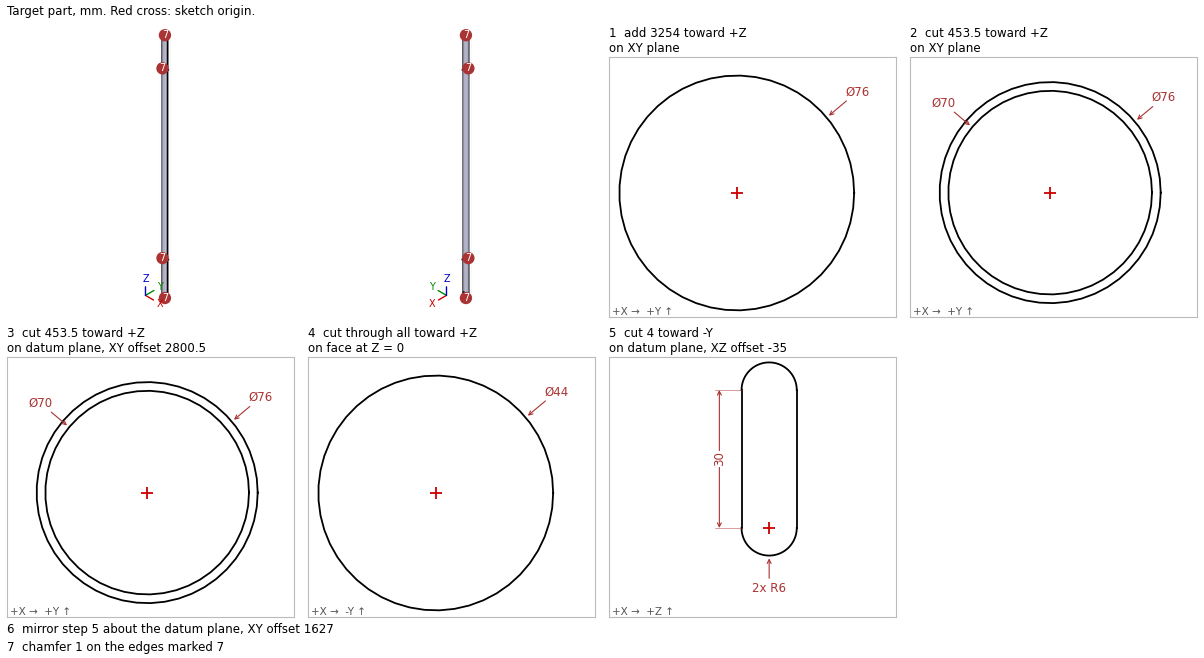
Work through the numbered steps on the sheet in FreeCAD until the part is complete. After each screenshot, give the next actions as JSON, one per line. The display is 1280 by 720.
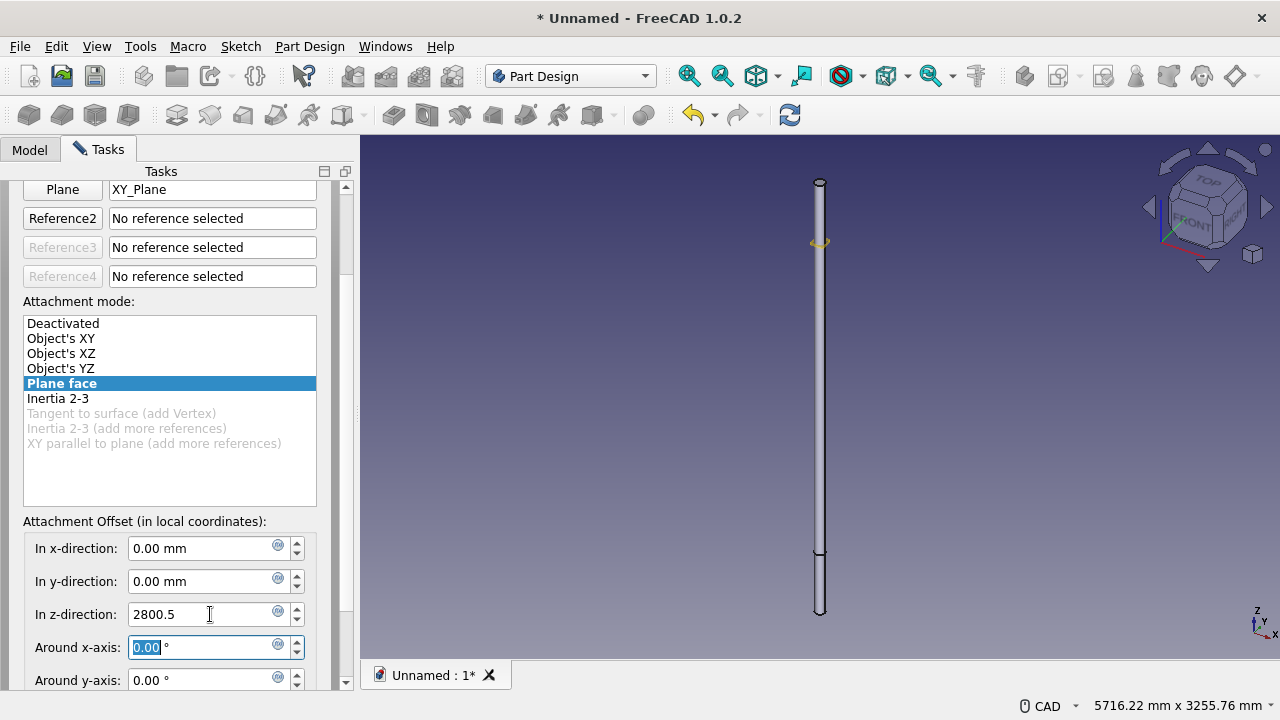
{"action": "scroll", "coordinate": [346, 436], "scroll_direction": "up", "scroll_amount": 3}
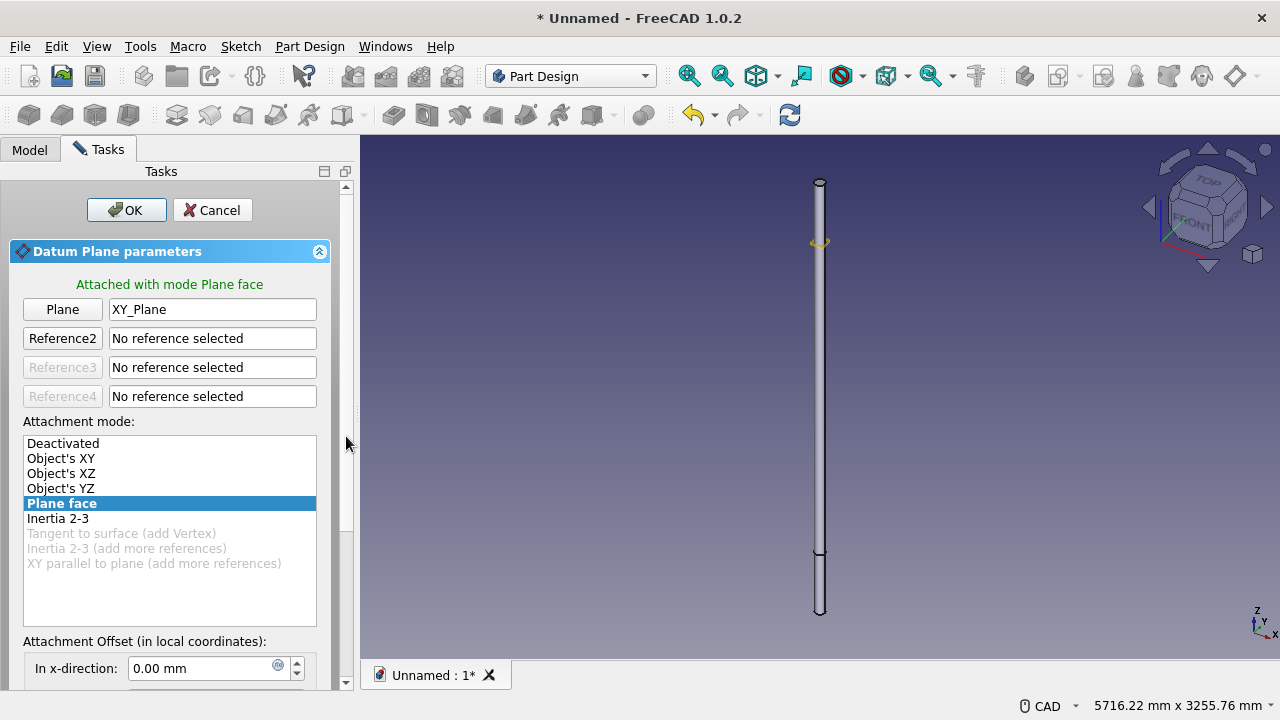
{"action": "left_click", "coordinate": [127, 210]}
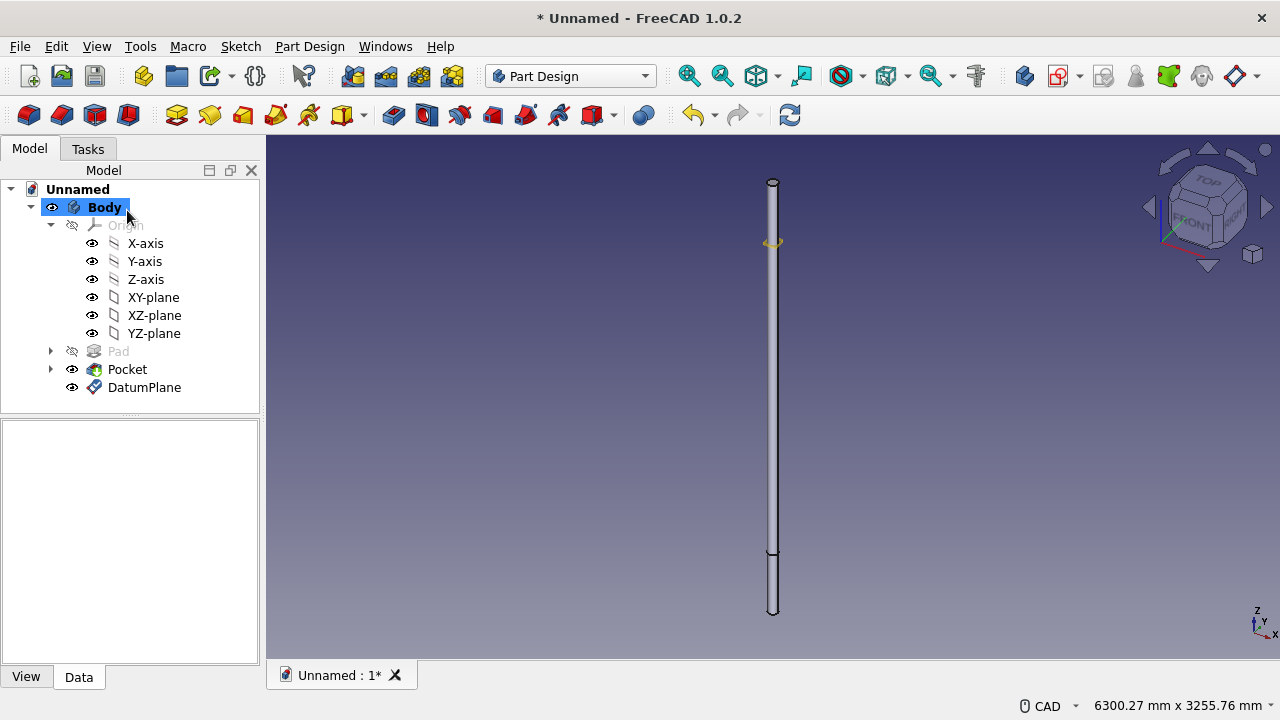
{"action": "left_click", "coordinate": [117, 387]}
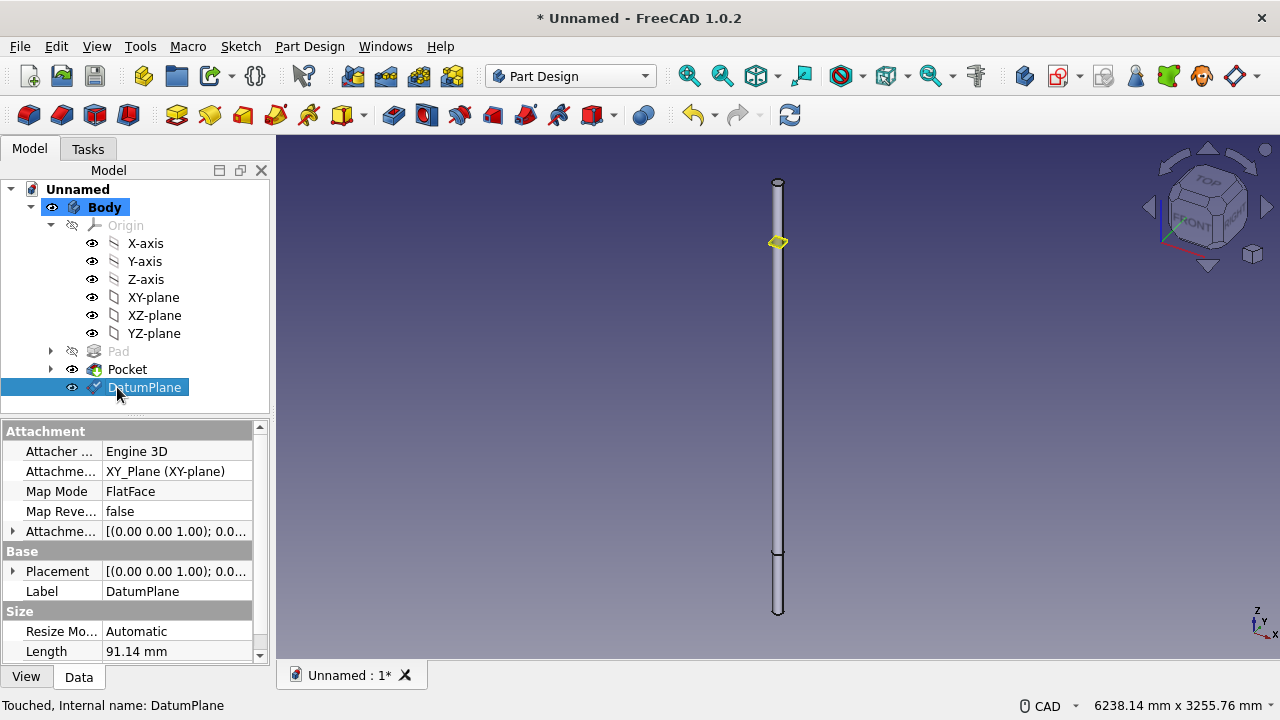
{"action": "left_click", "coordinate": [1058, 76]}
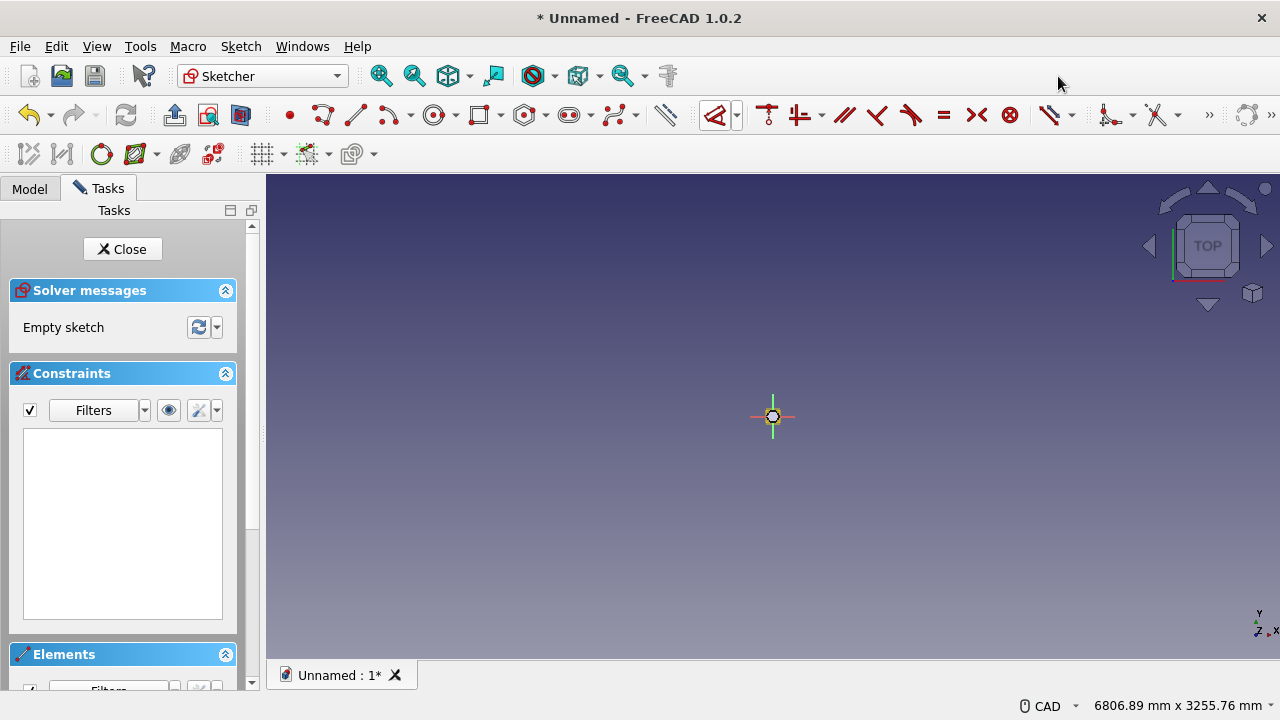
{"action": "left_click", "coordinate": [241, 116]}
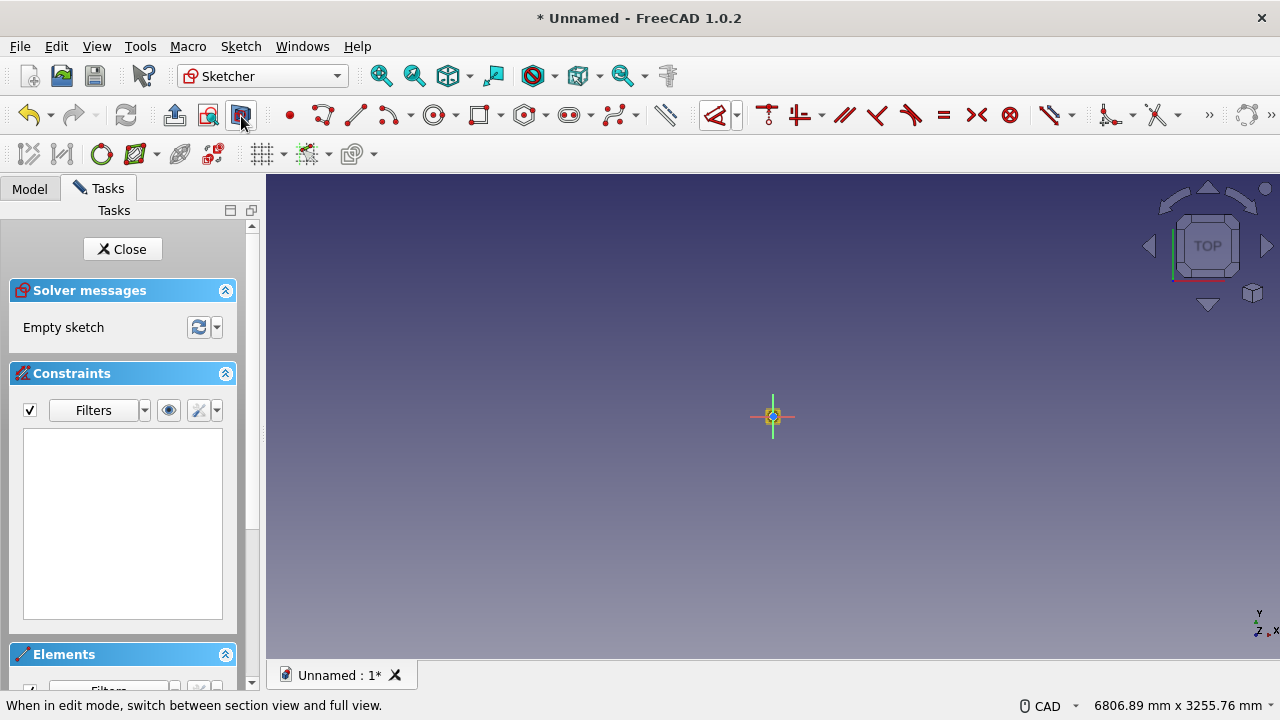
{"action": "scroll", "coordinate": [777, 416], "scroll_direction": "up", "scroll_amount": 15}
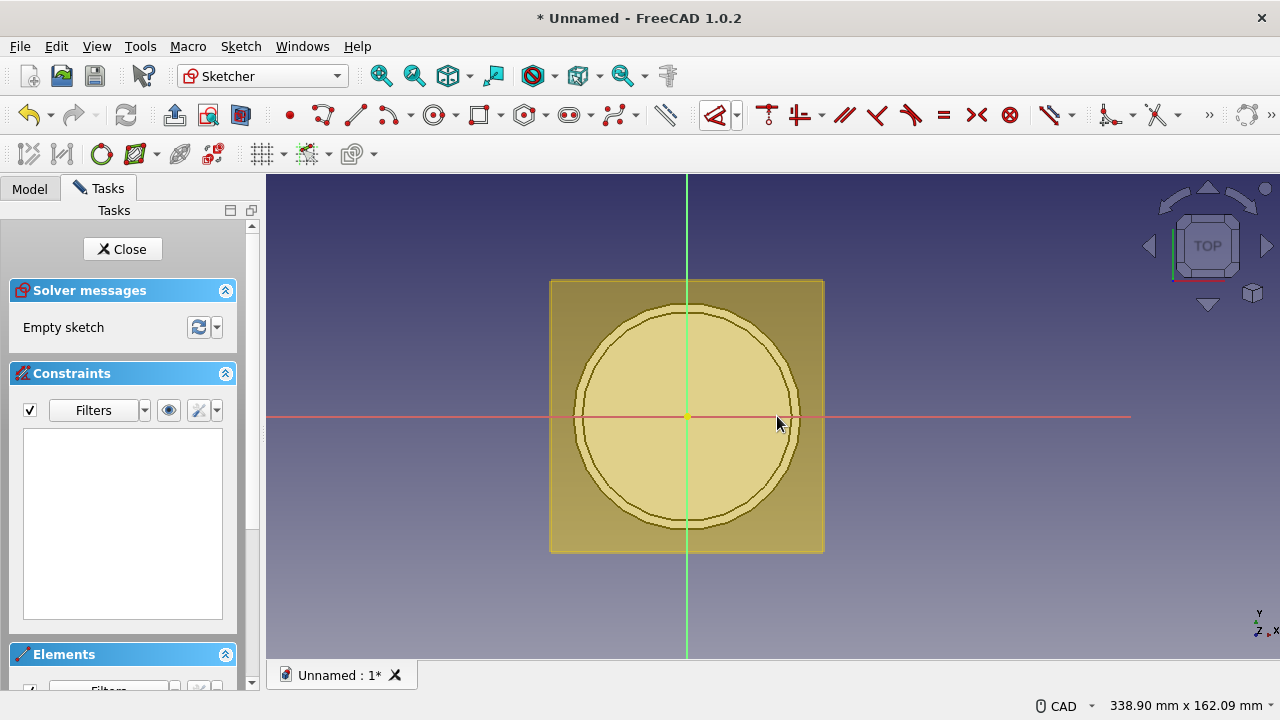
{"action": "left_click", "coordinate": [434, 116]}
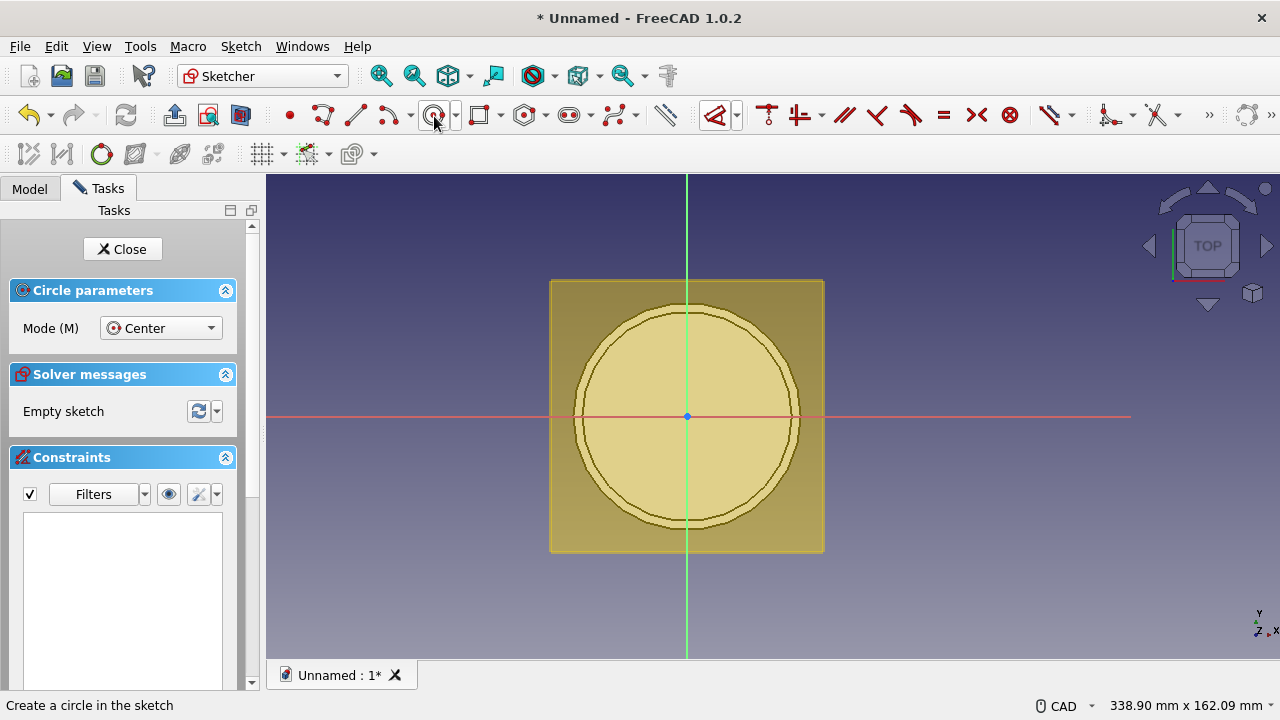
{"action": "left_click", "coordinate": [687, 416]}
{"action": "left_click", "coordinate": [767, 336]}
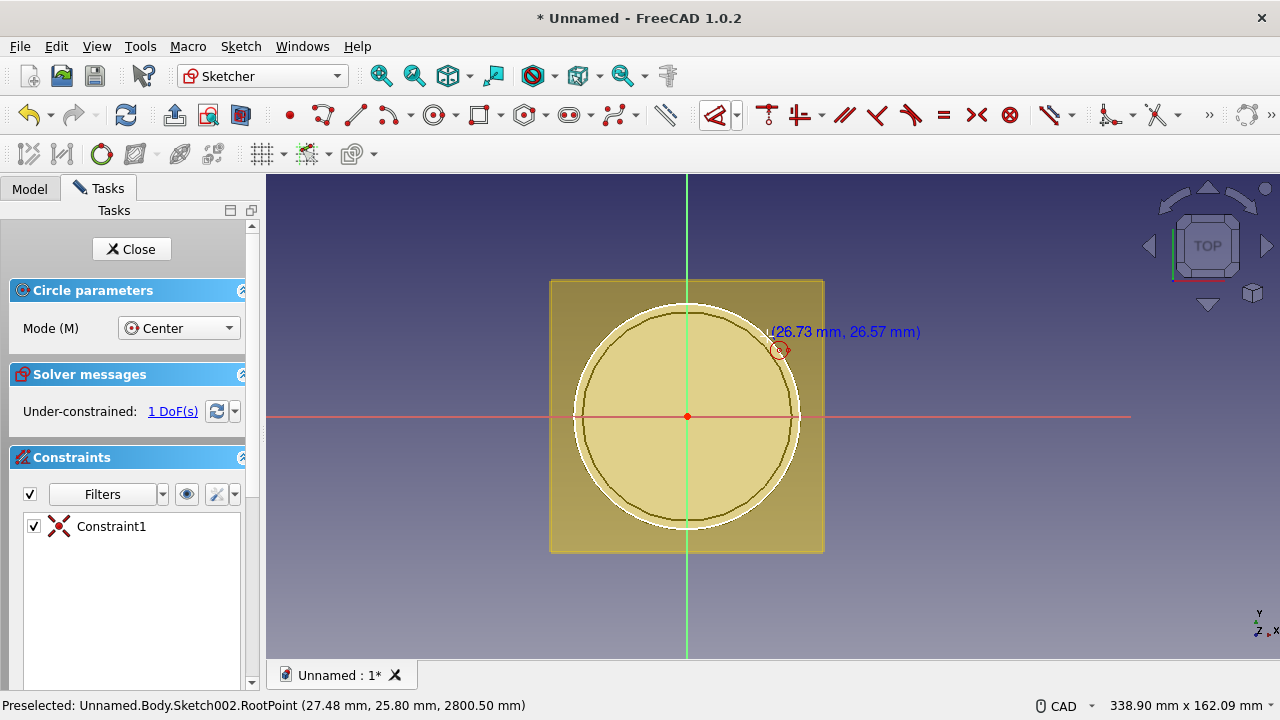
{"action": "left_click", "coordinate": [687, 416]}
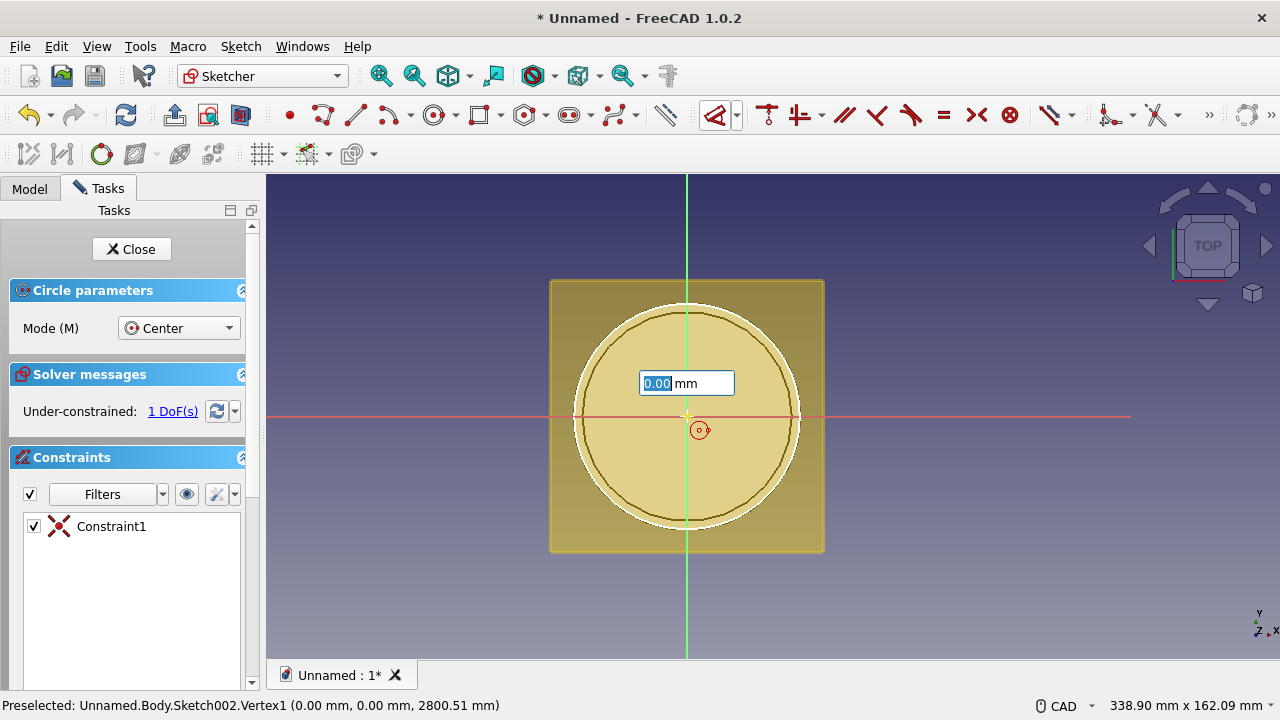
{"action": "scroll", "coordinate": [761, 342], "scroll_direction": "up", "scroll_amount": 3}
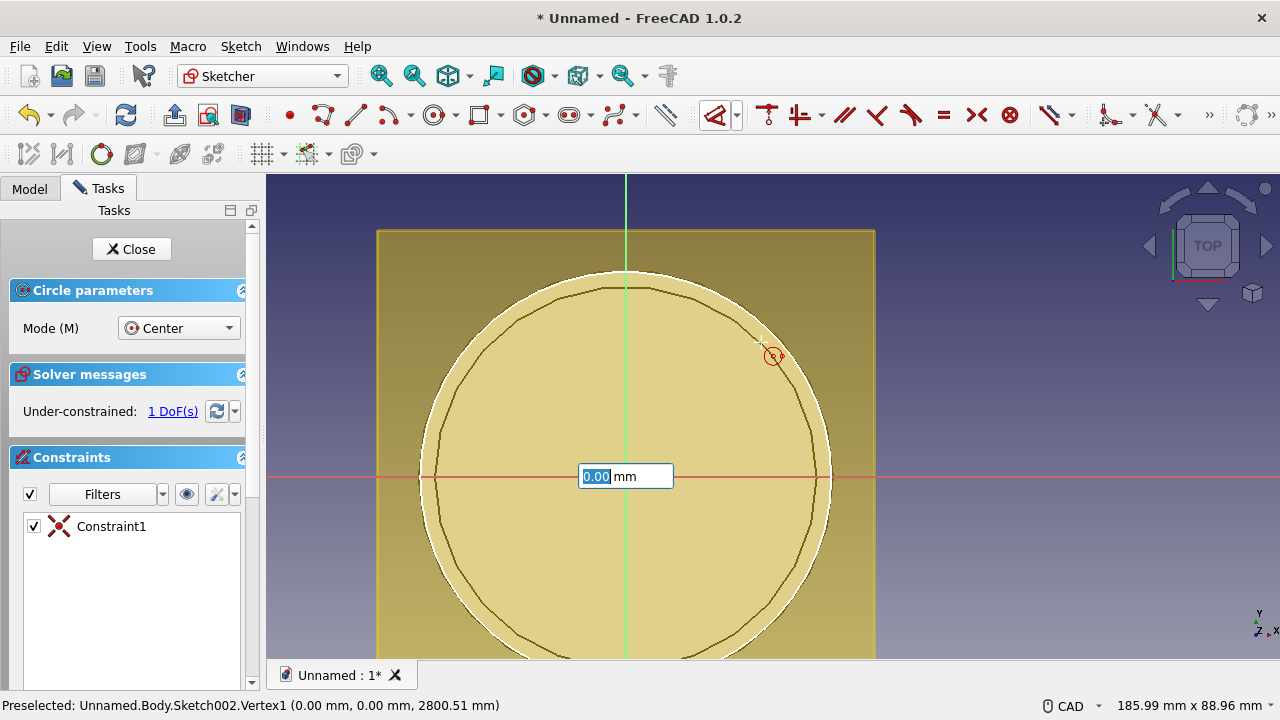
{"action": "left_click", "coordinate": [761, 343]}
{"action": "key", "text": "Escape"}